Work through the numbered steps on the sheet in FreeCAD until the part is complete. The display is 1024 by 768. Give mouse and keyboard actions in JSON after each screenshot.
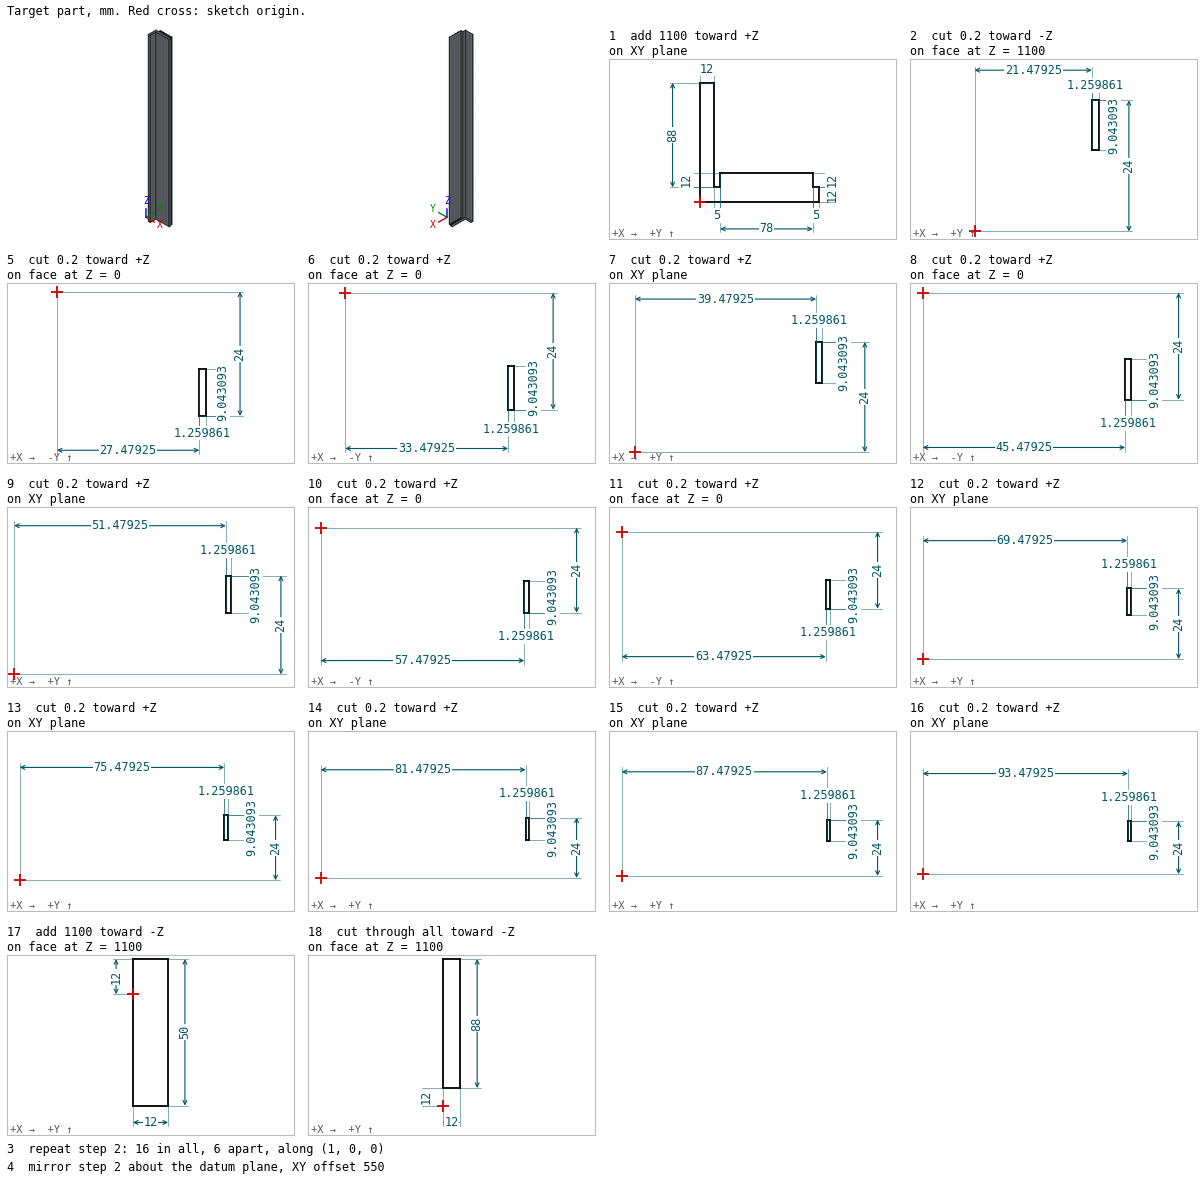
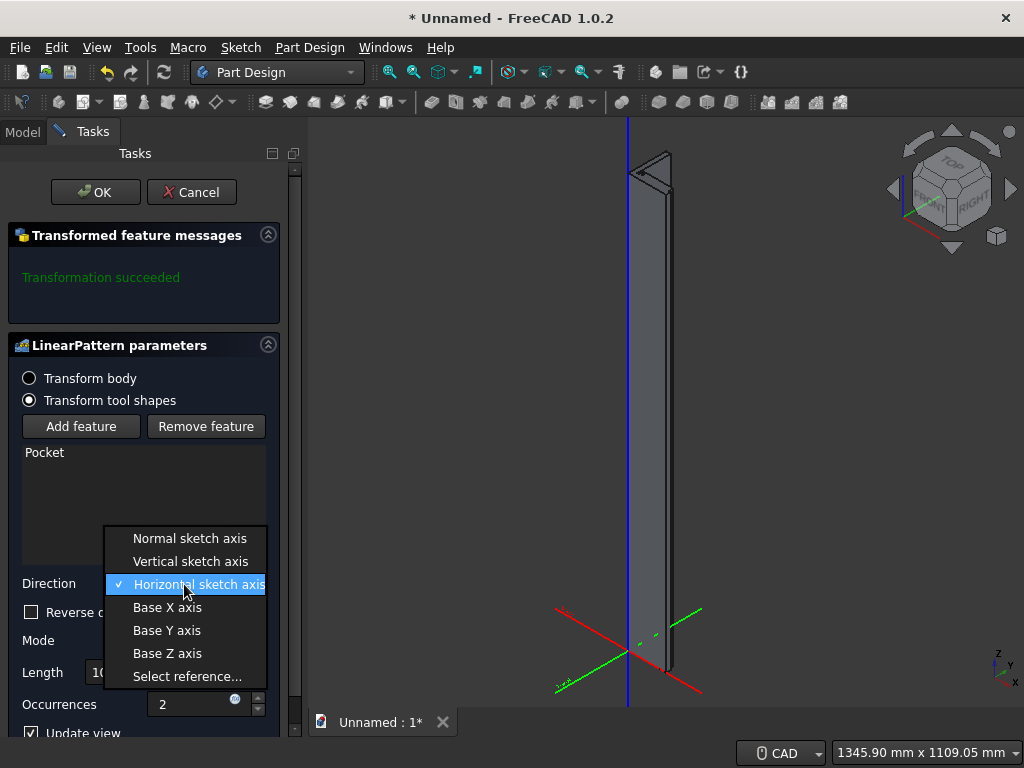
{"action": "left_click", "coordinate": [184, 608]}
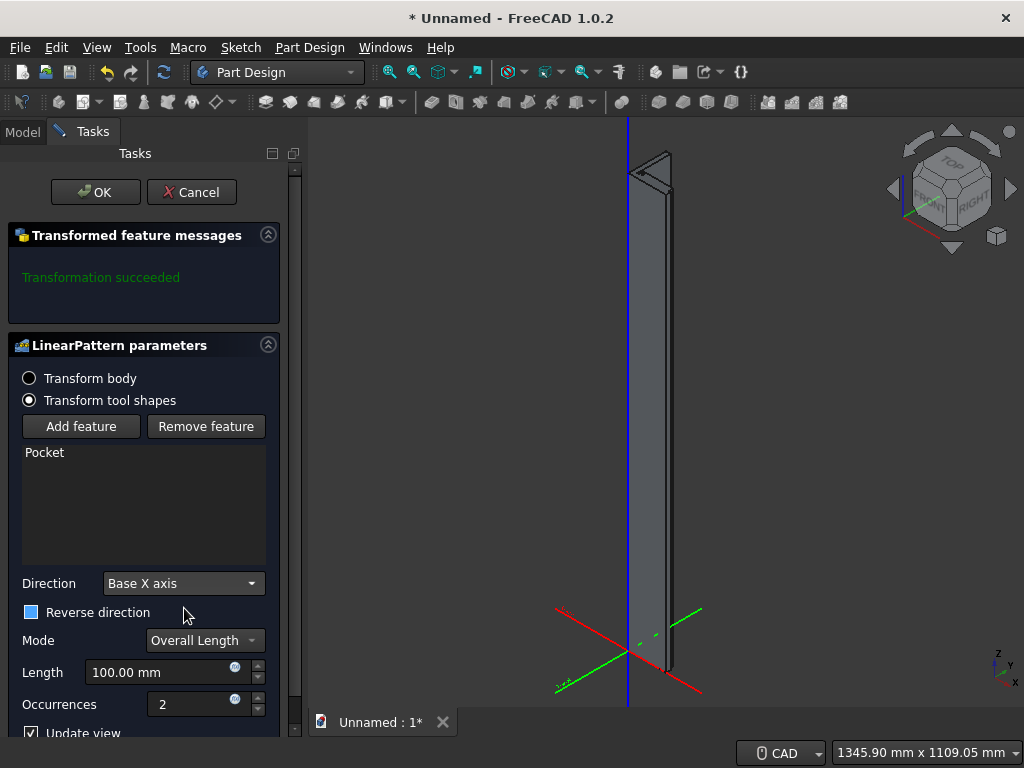
{"action": "left_click", "coordinate": [206, 640]}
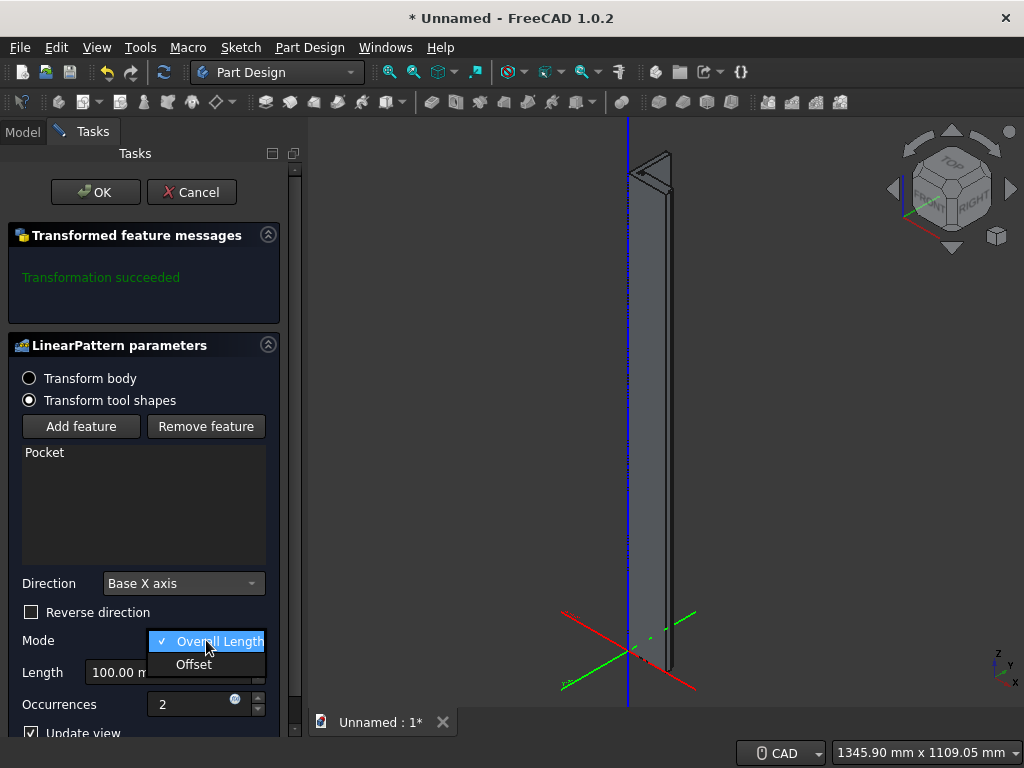
{"action": "left_click", "coordinate": [206, 664]}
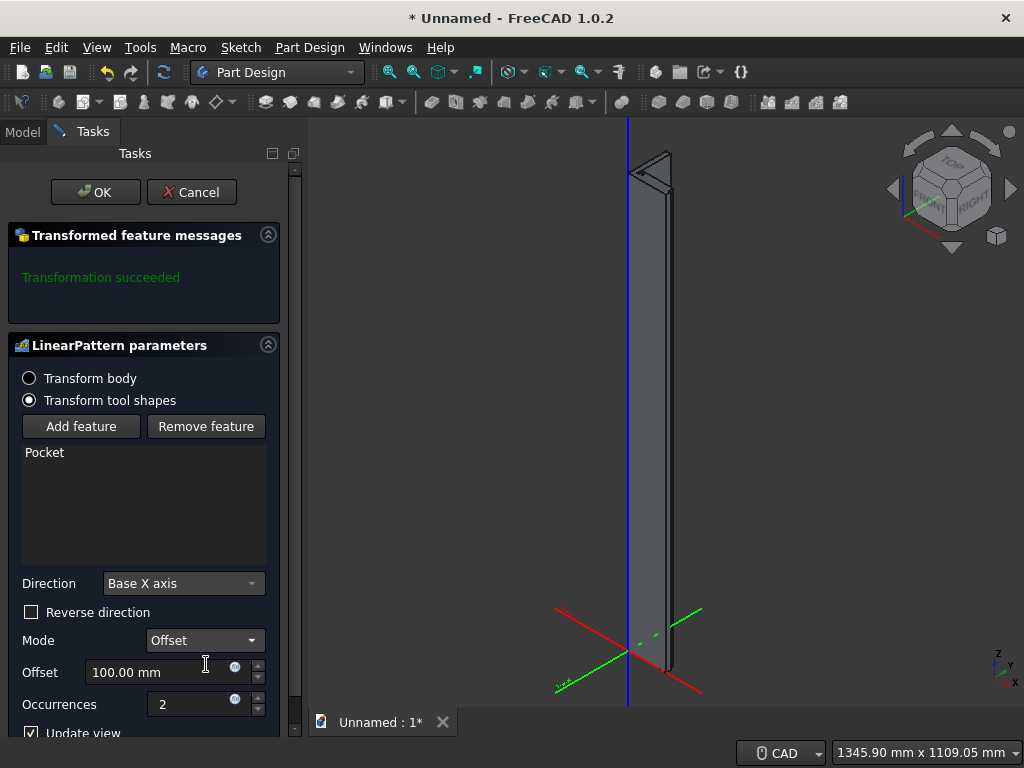
{"action": "triple_click", "coordinate": [168, 672]}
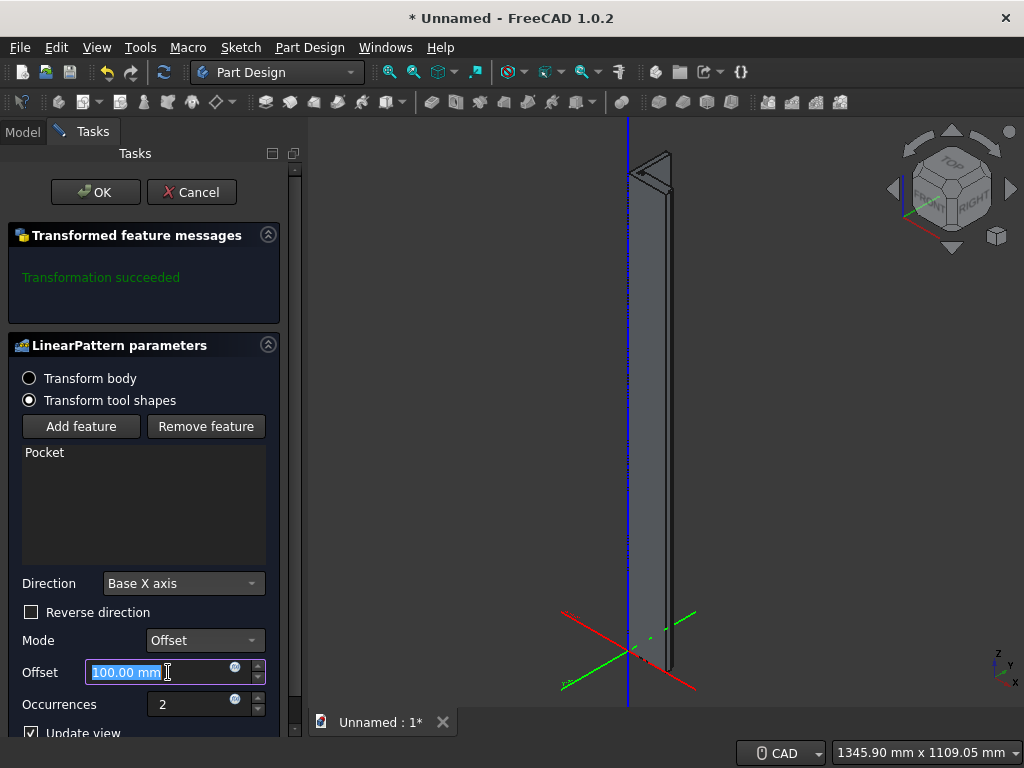
{"action": "type", "text": "6"}
{"action": "key", "text": "Tab"}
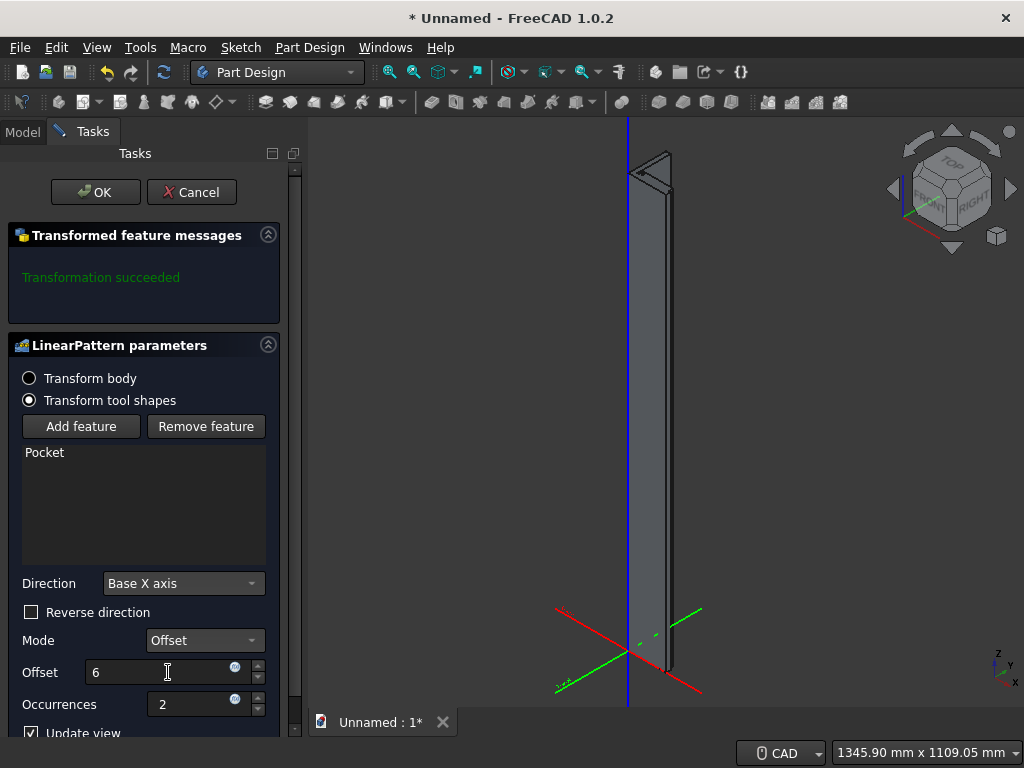
{"action": "triple_click", "coordinate": [198, 704]}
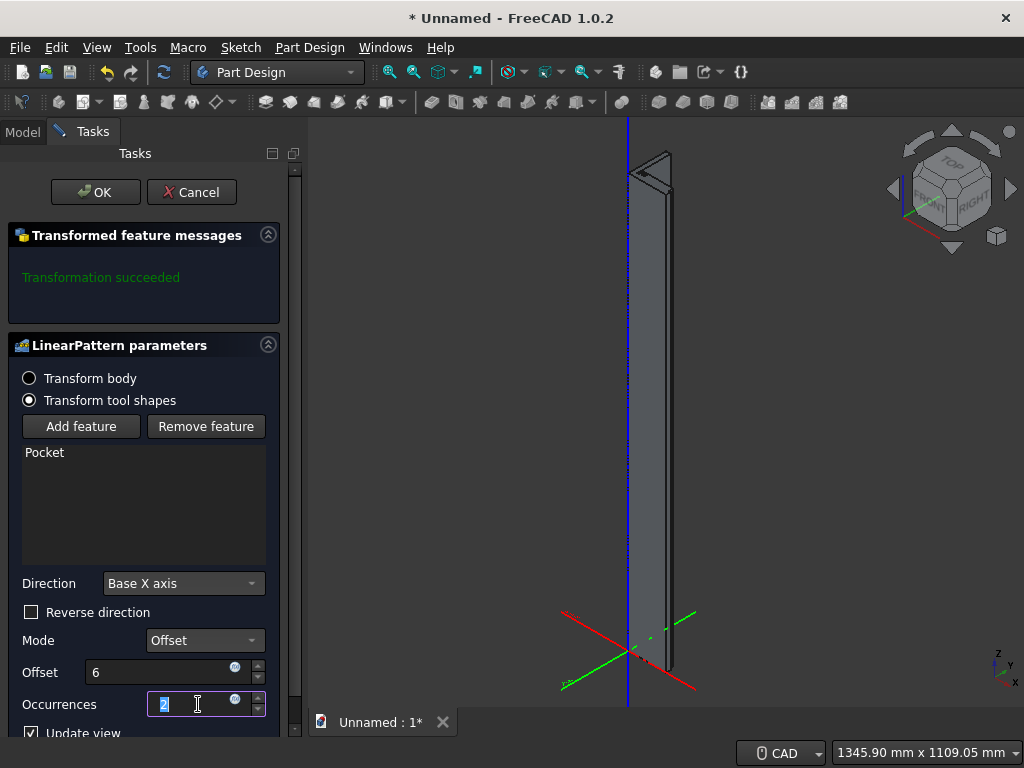
{"action": "type", "text": "16"}
{"action": "key", "text": "Tab"}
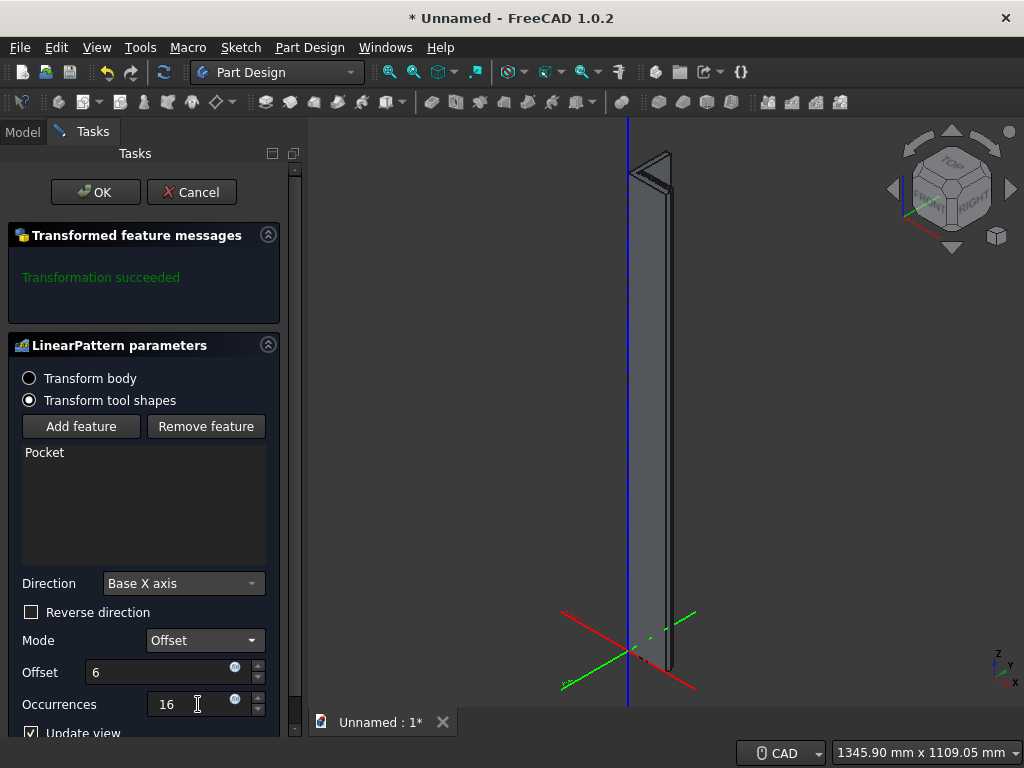
{"action": "left_click", "coordinate": [96, 192]}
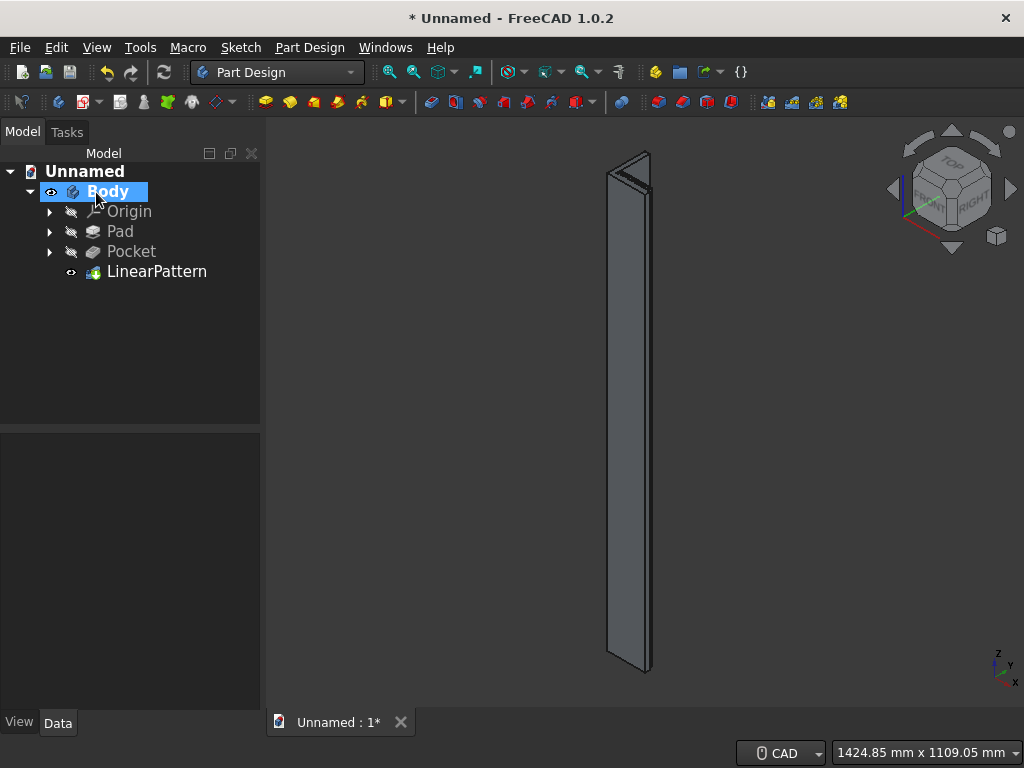
{"action": "left_click", "coordinate": [50, 212]}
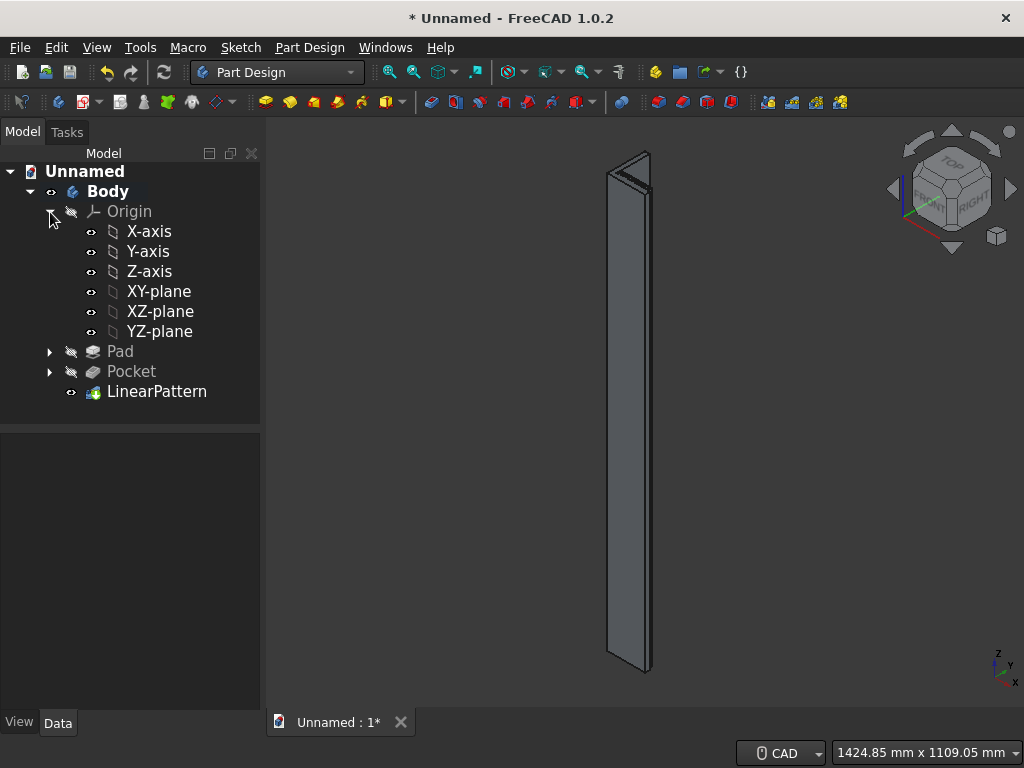
{"action": "left_click", "coordinate": [136, 292]}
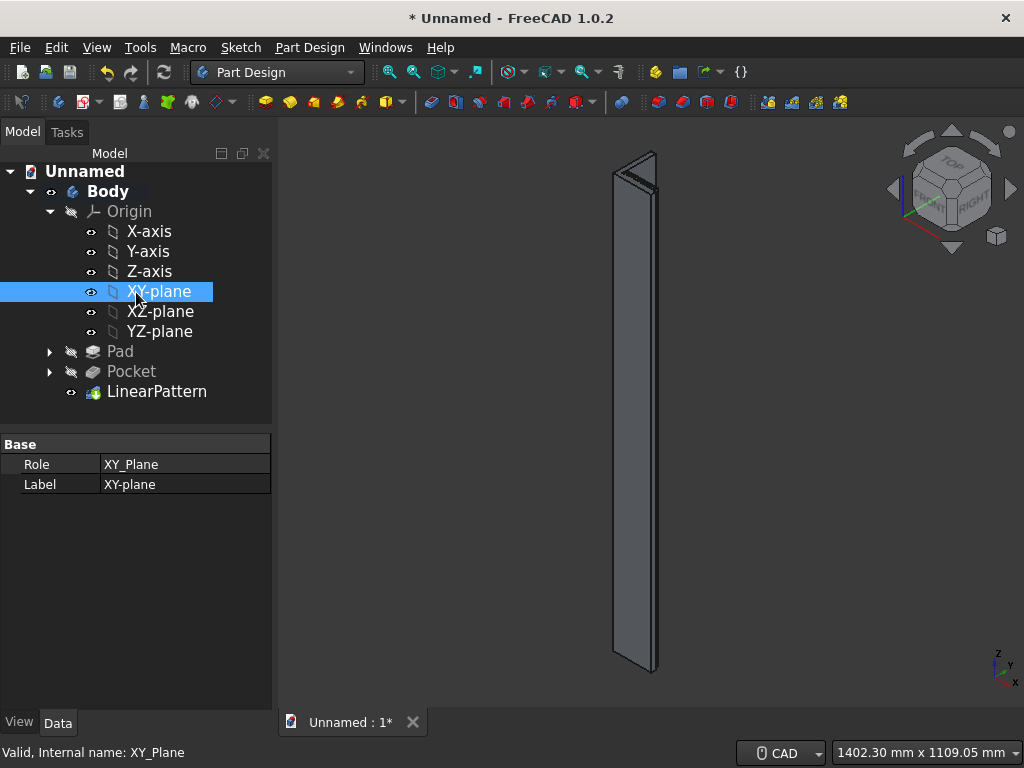
{"action": "left_click", "coordinate": [216, 102]}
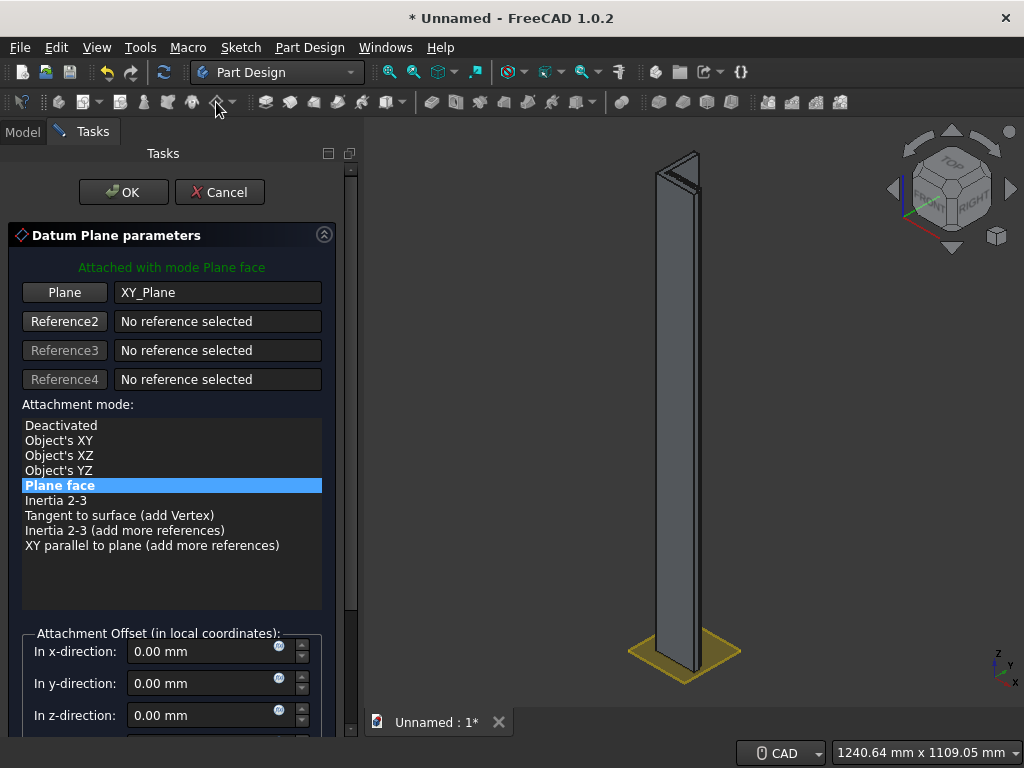
{"action": "triple_click", "coordinate": [210, 715]}